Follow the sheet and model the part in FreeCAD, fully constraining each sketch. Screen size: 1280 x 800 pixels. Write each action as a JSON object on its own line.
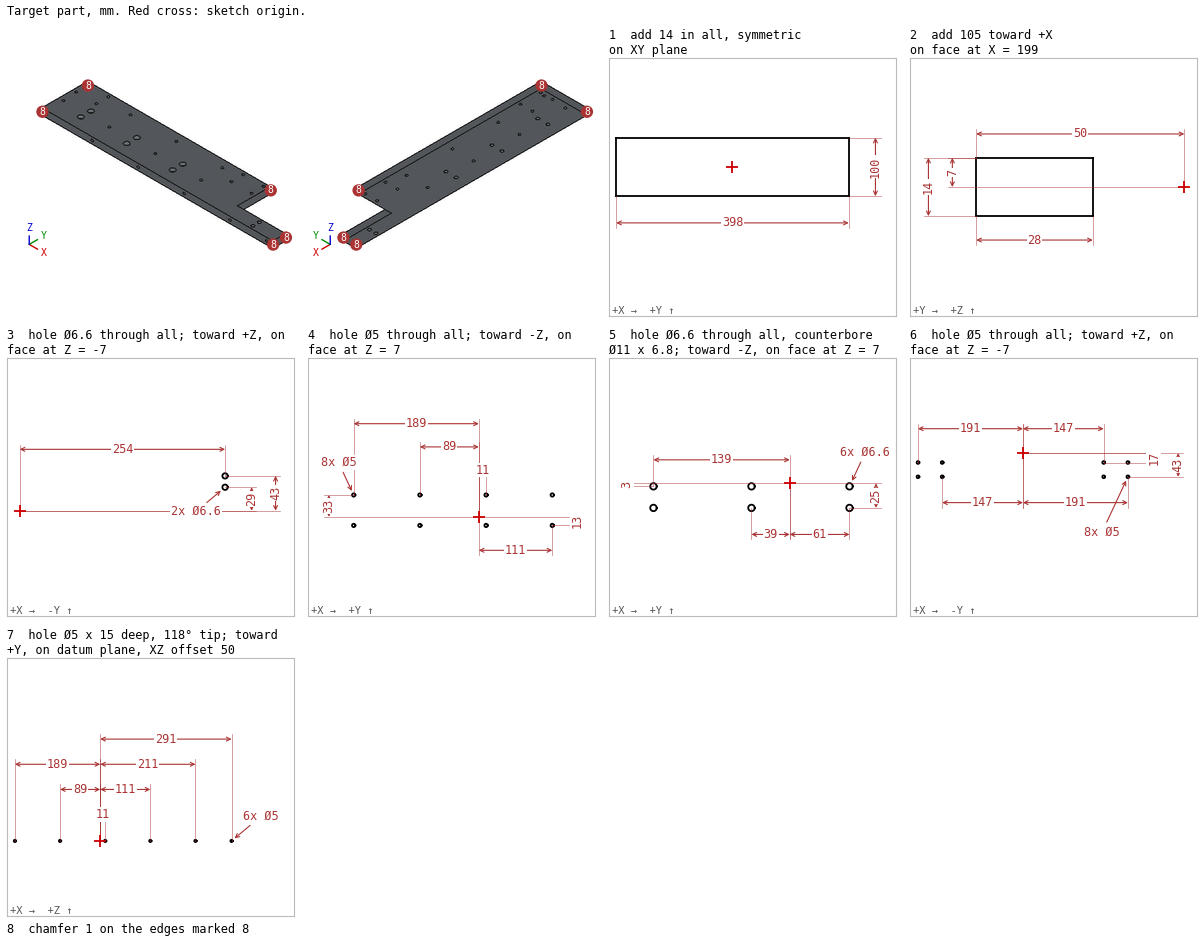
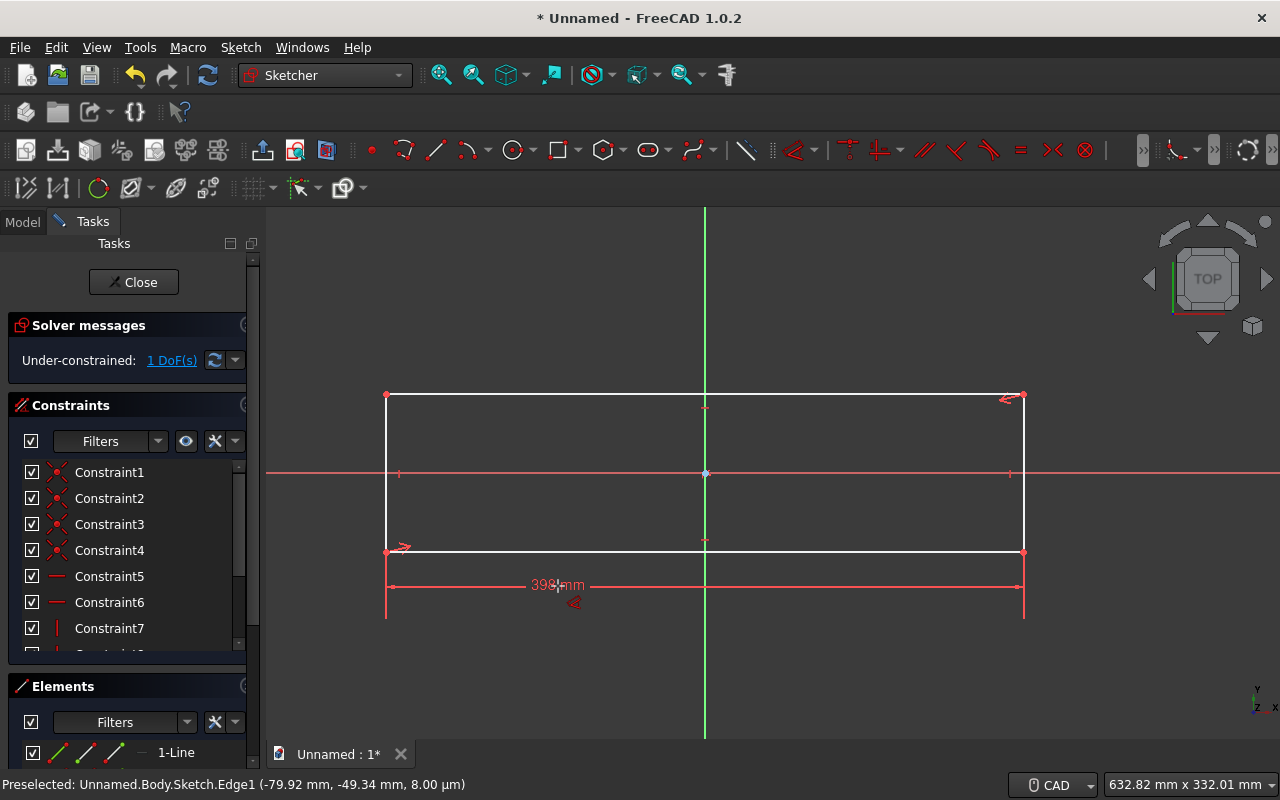
{"action": "left_click", "coordinate": [1024, 505]}
{"action": "left_click", "coordinate": [1058, 437]}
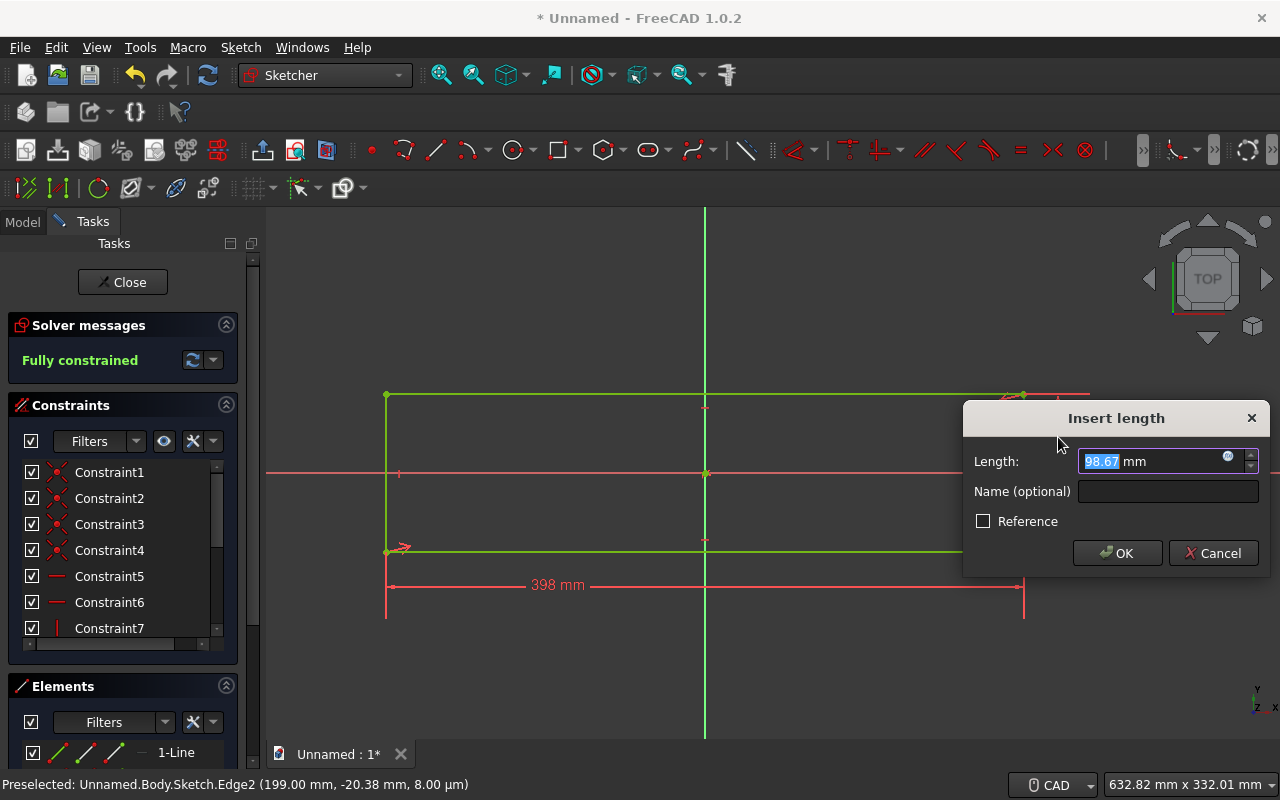
{"action": "type", "text": "100"}
{"action": "key", "text": "Return"}
{"action": "key", "text": "Escape"}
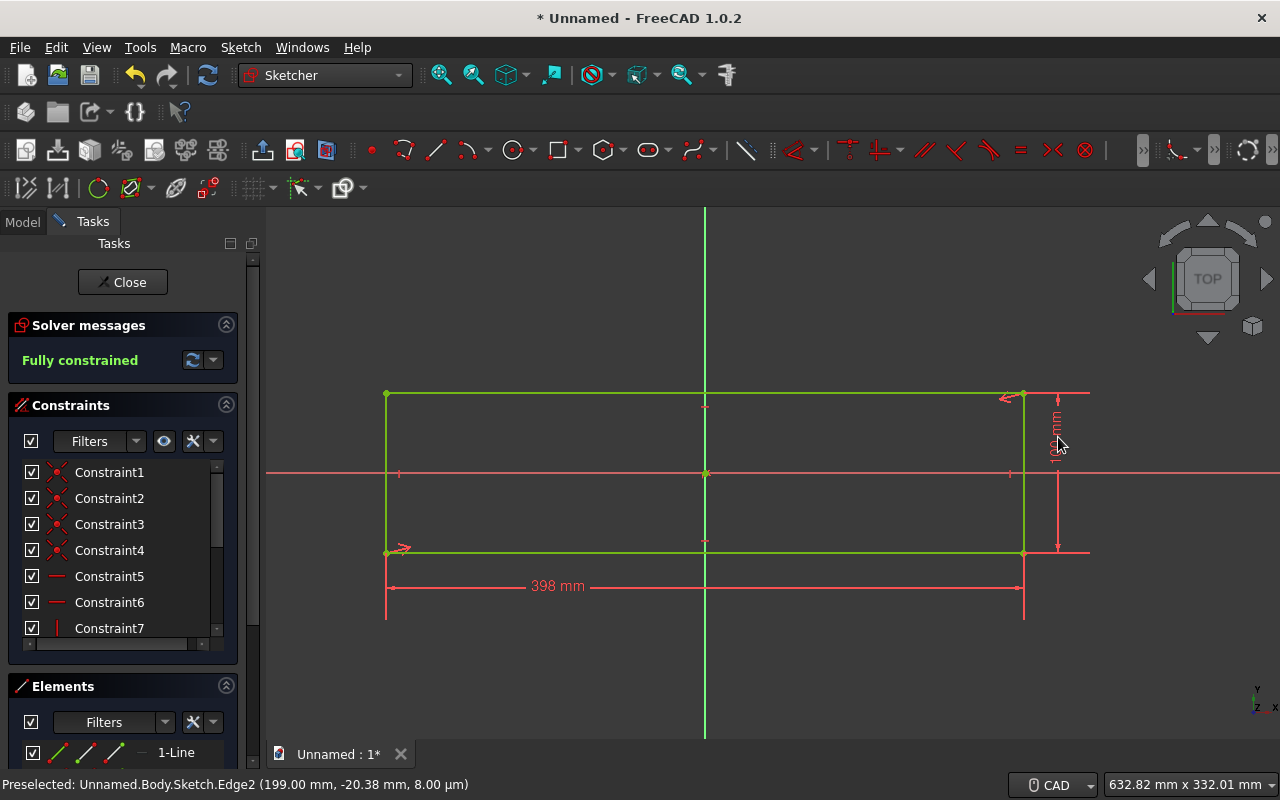
{"action": "left_click", "coordinate": [123, 282]}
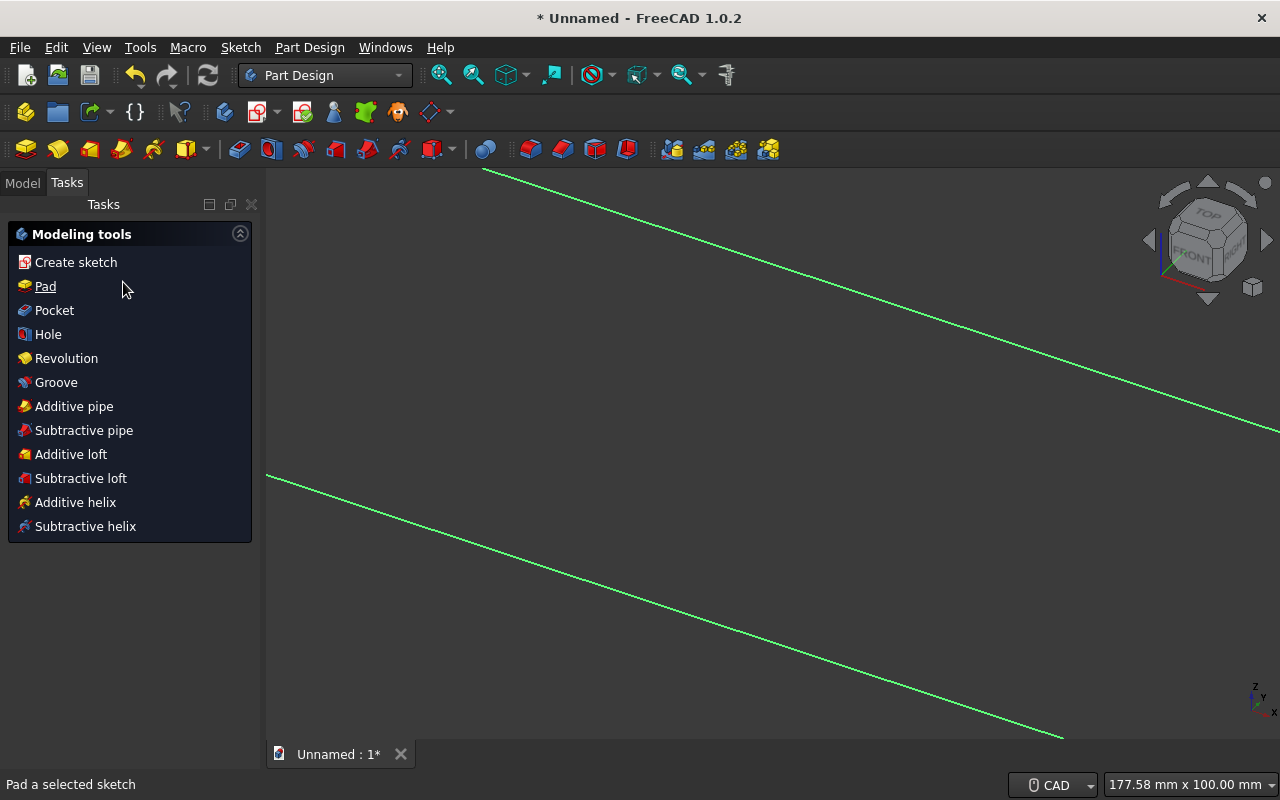
{"action": "left_click", "coordinate": [26, 150]}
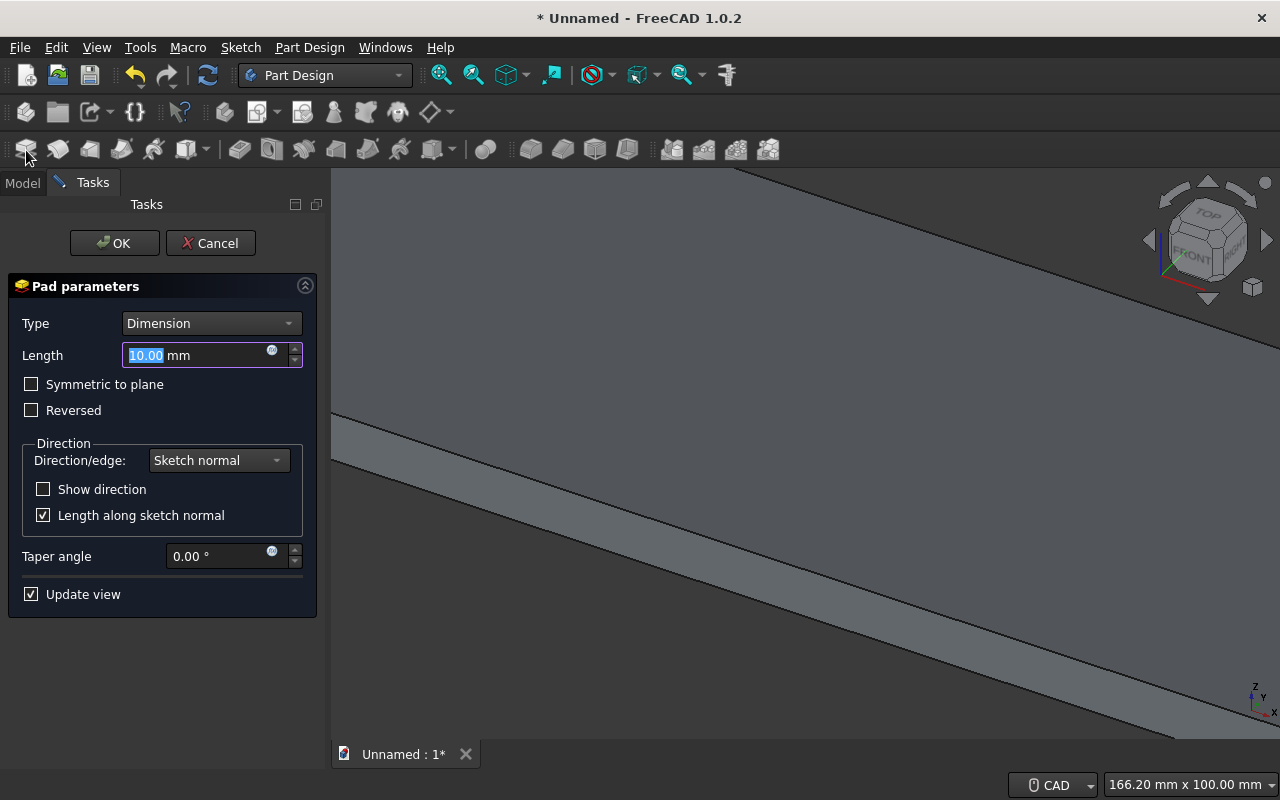
{"action": "type", "text": "14"}
{"action": "key", "text": "Tab"}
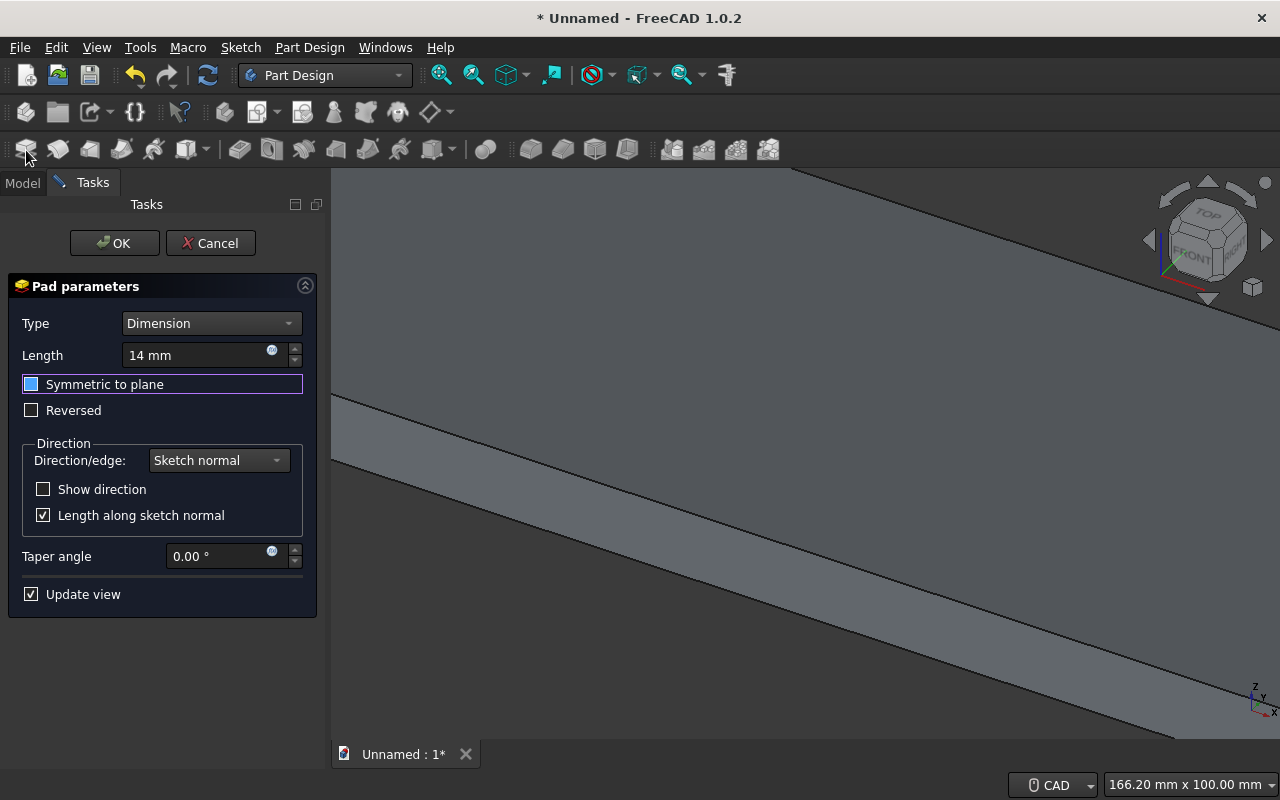
{"action": "left_click", "coordinate": [30, 384]}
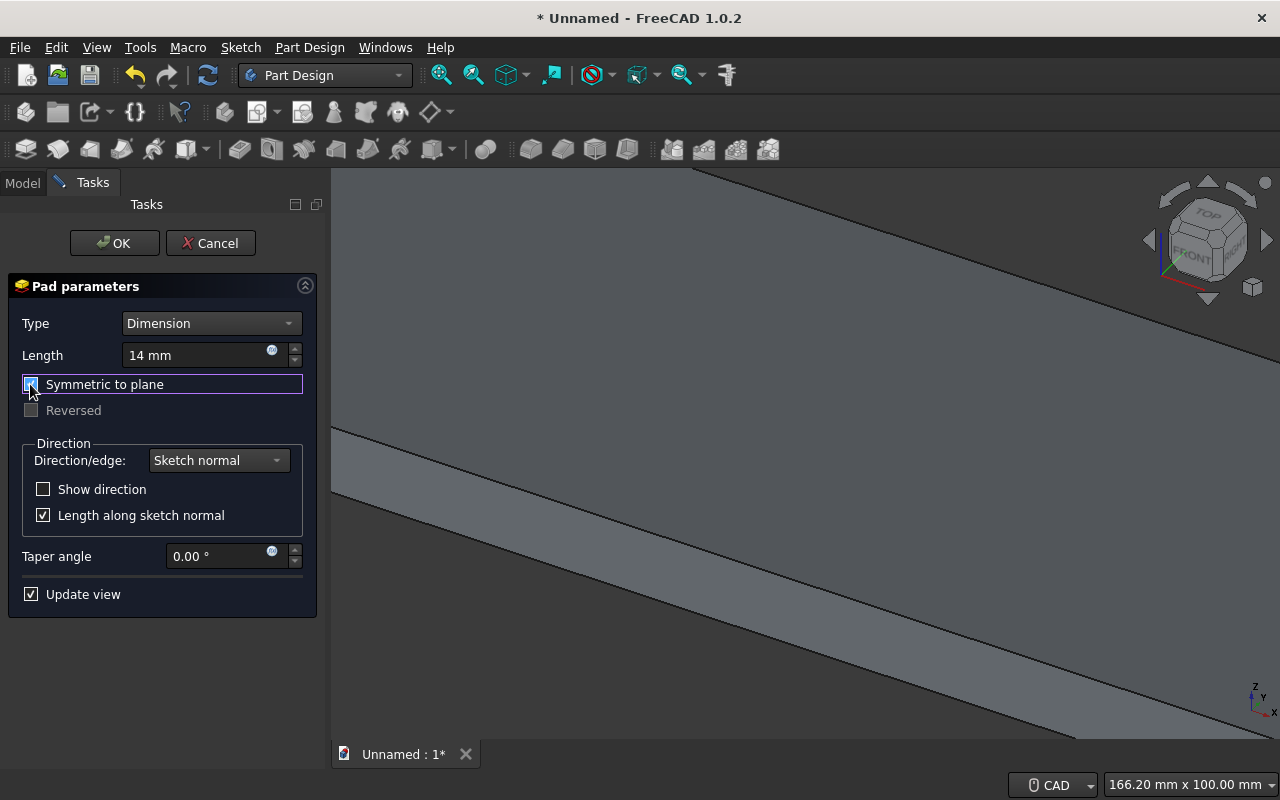
{"action": "left_click", "coordinate": [115, 243]}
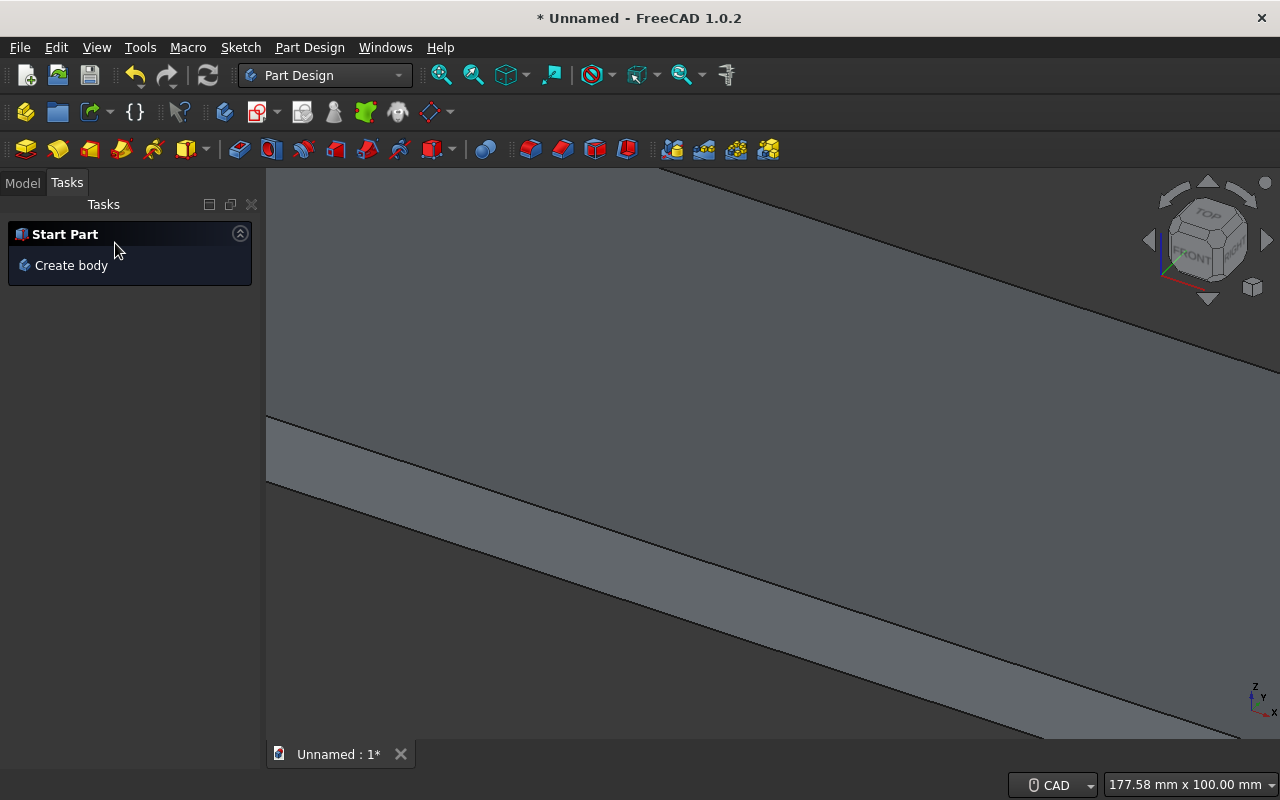
{"action": "key", "text": "v f"}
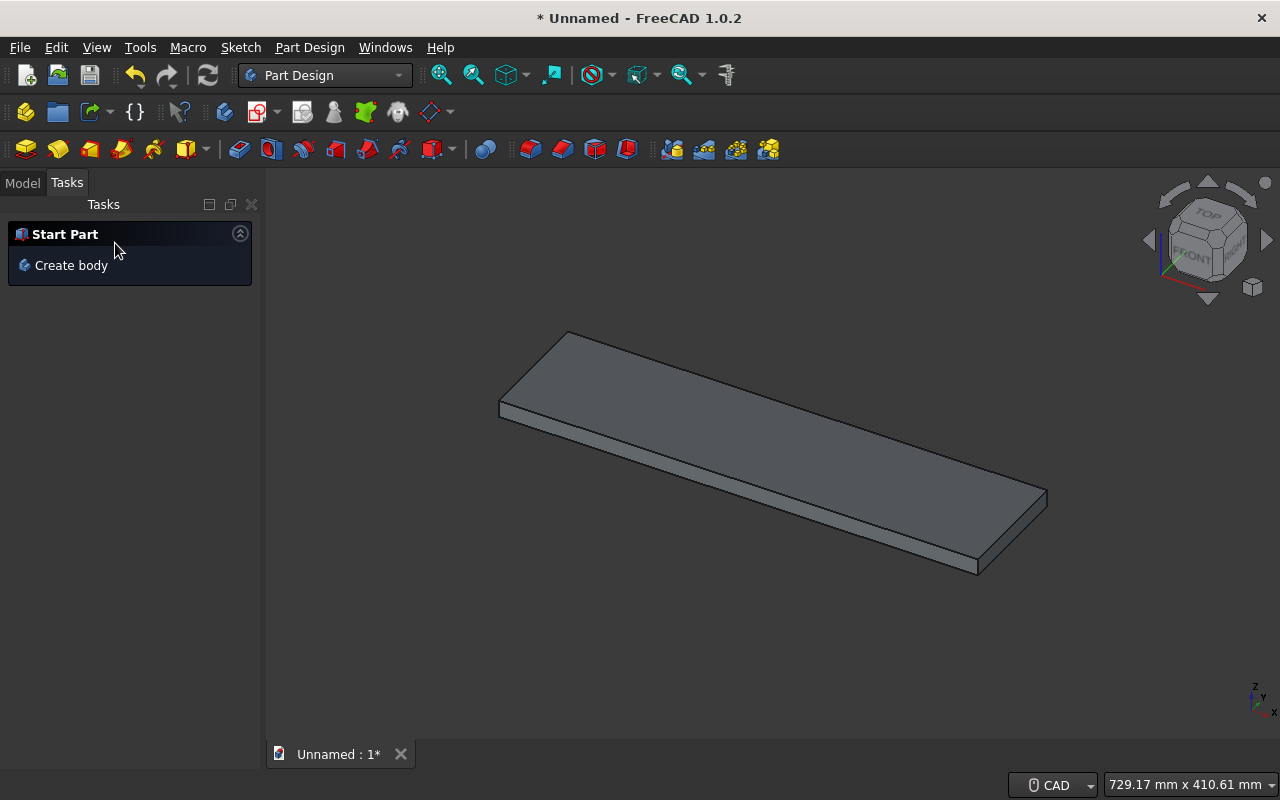
{"action": "key", "text": "0"}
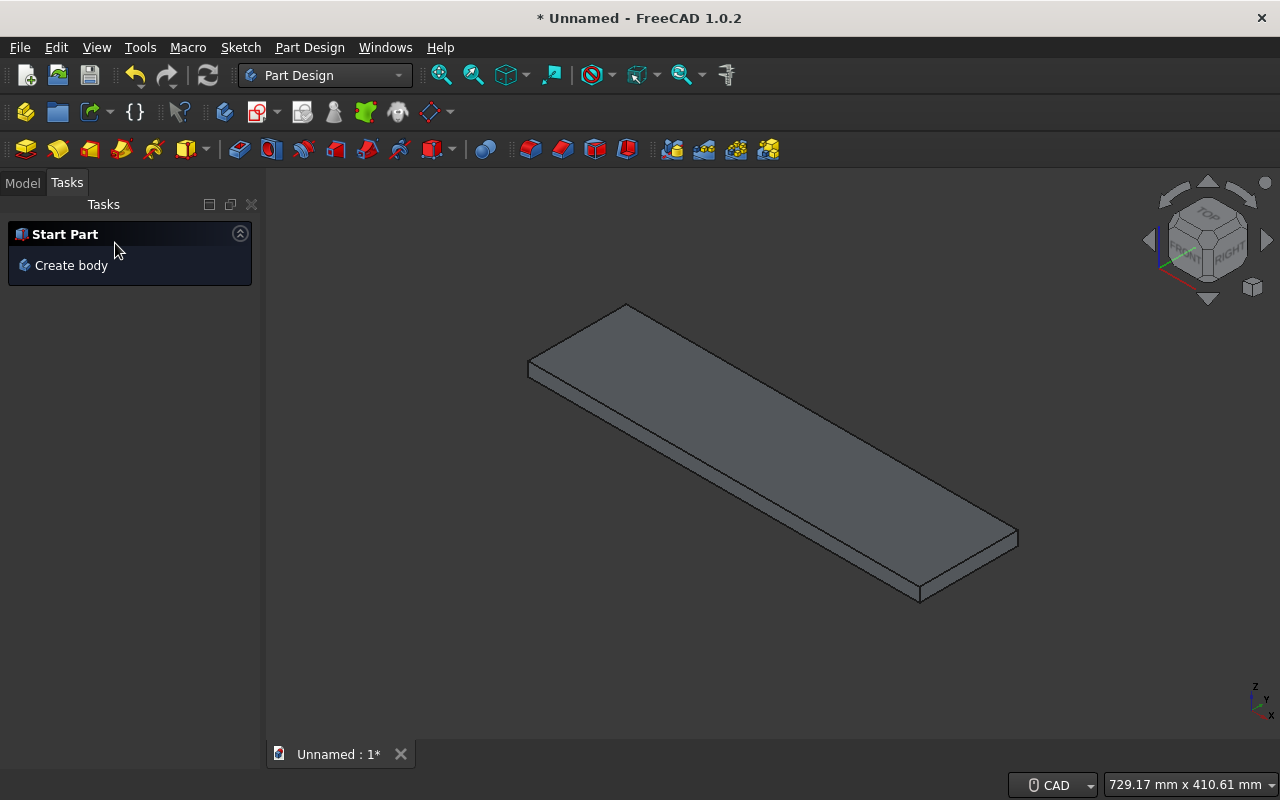
{"action": "key", "text": "3"}